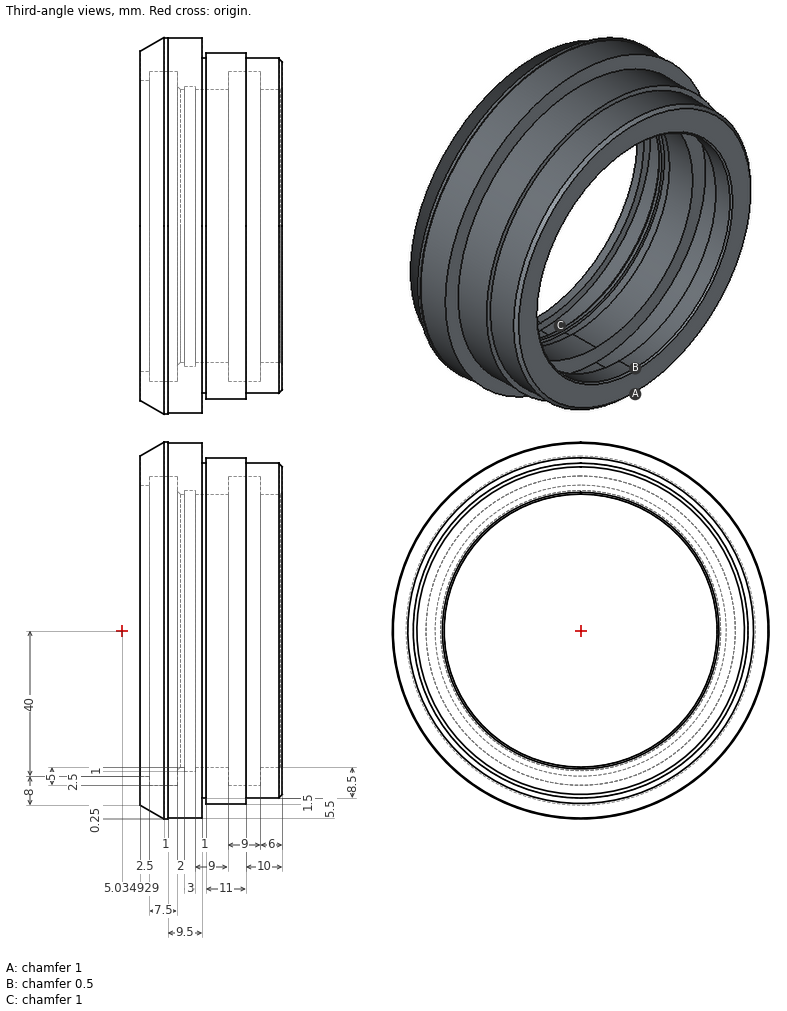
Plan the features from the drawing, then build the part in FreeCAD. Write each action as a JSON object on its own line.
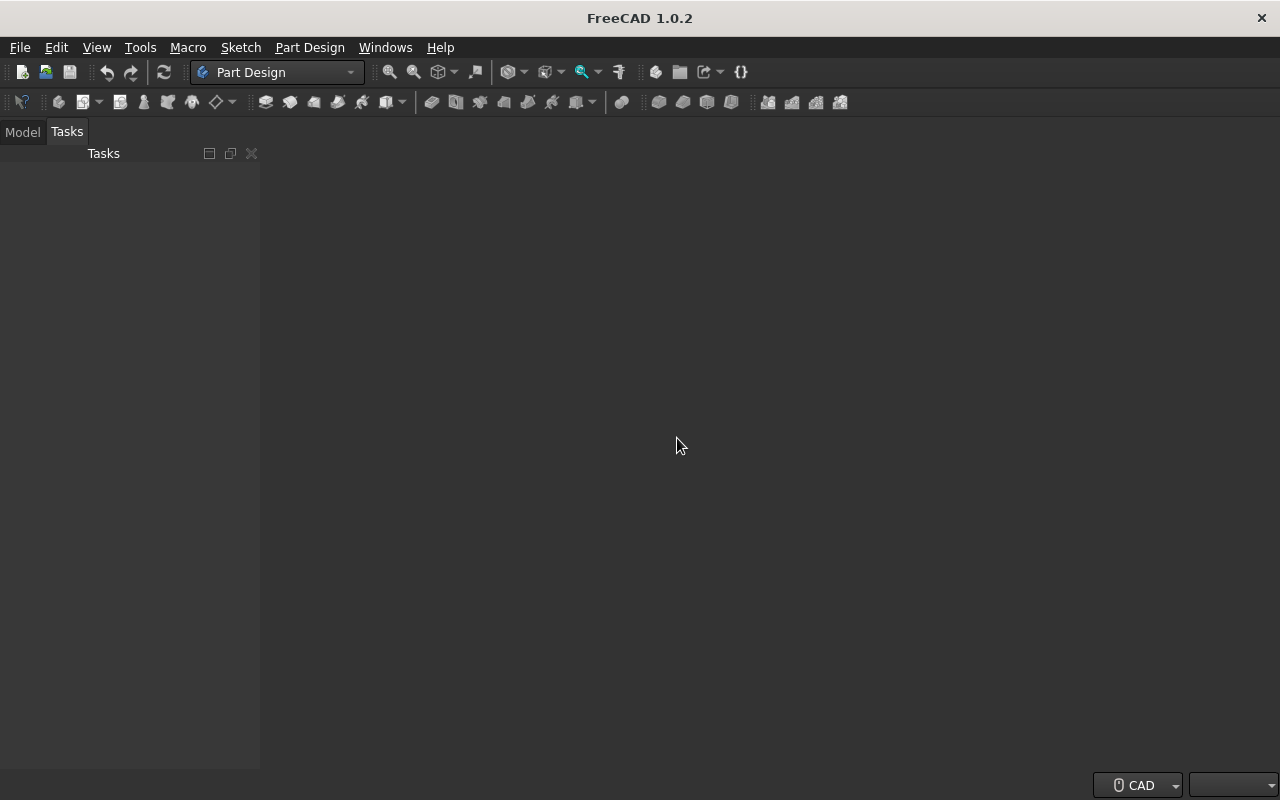
{"action": "key", "text": "ctrl+n"}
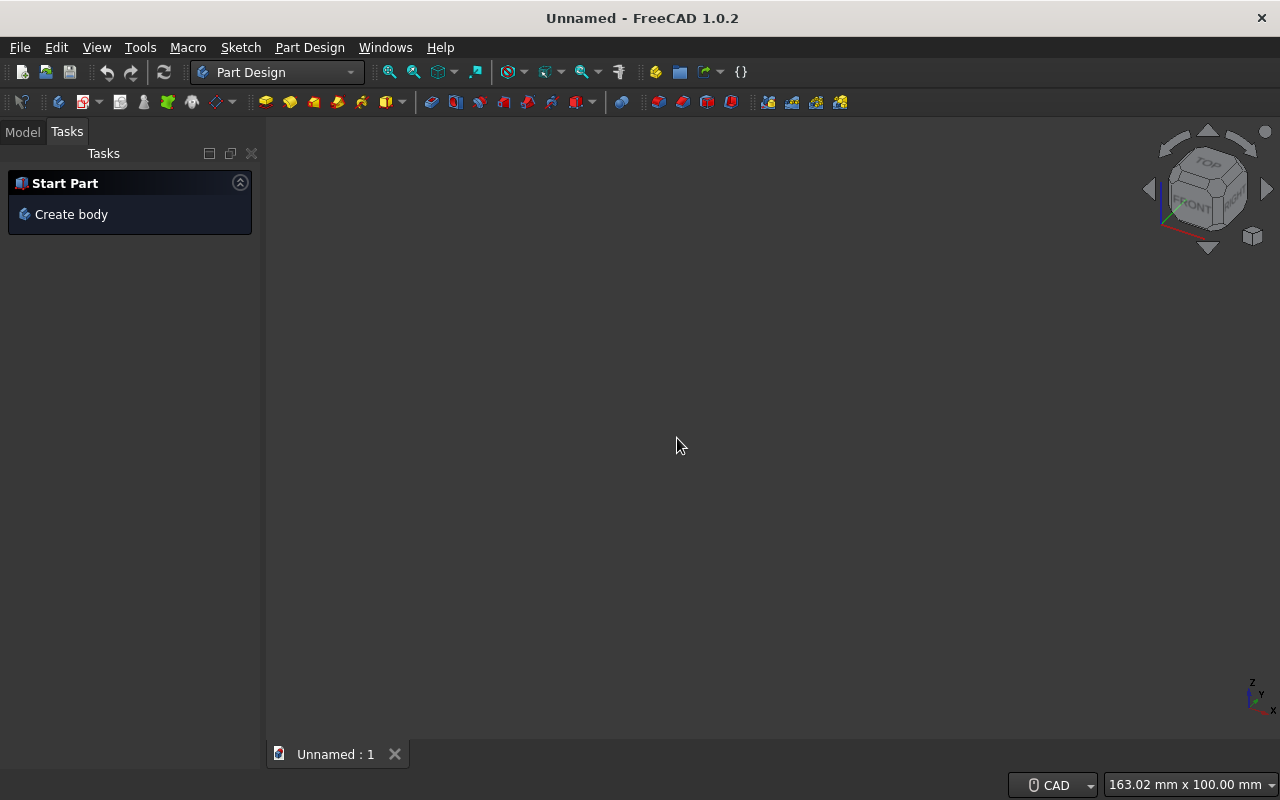
{"action": "left_click", "coordinate": [84, 102]}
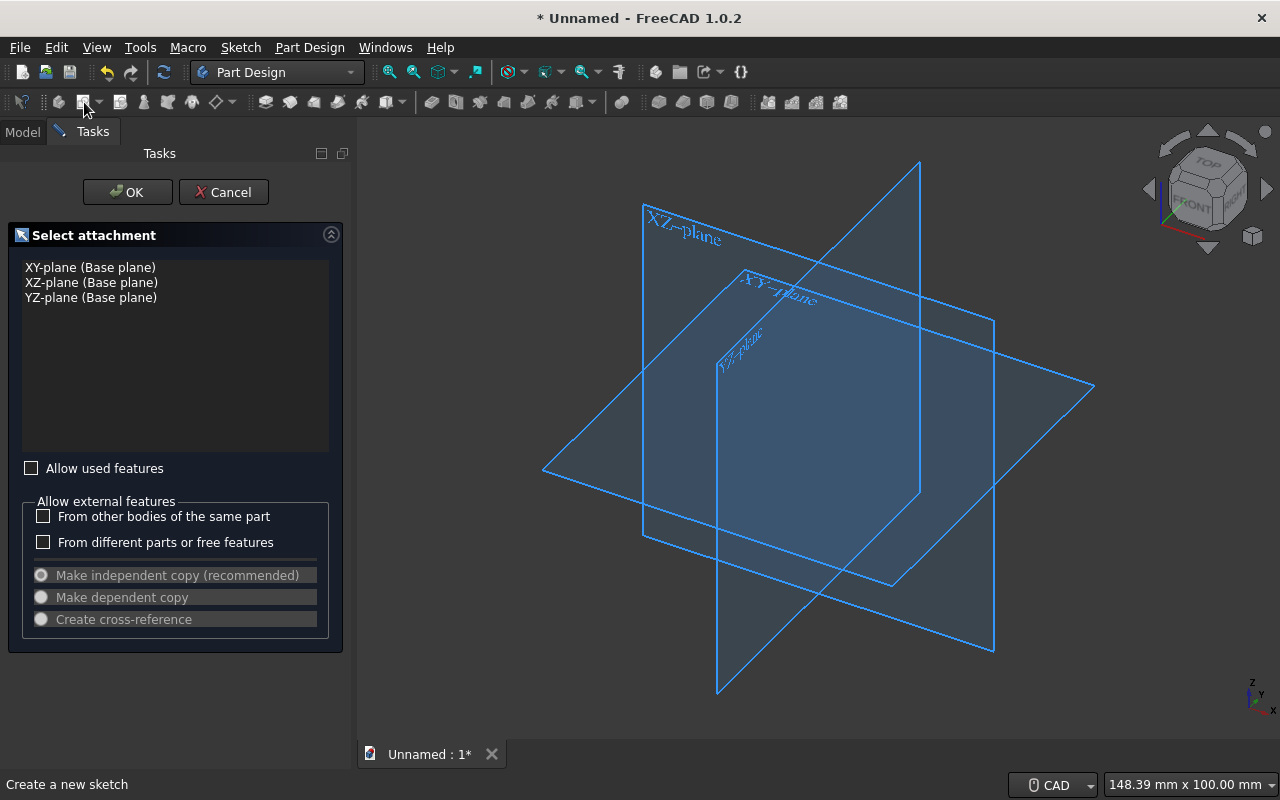
{"action": "left_click", "coordinate": [82, 282]}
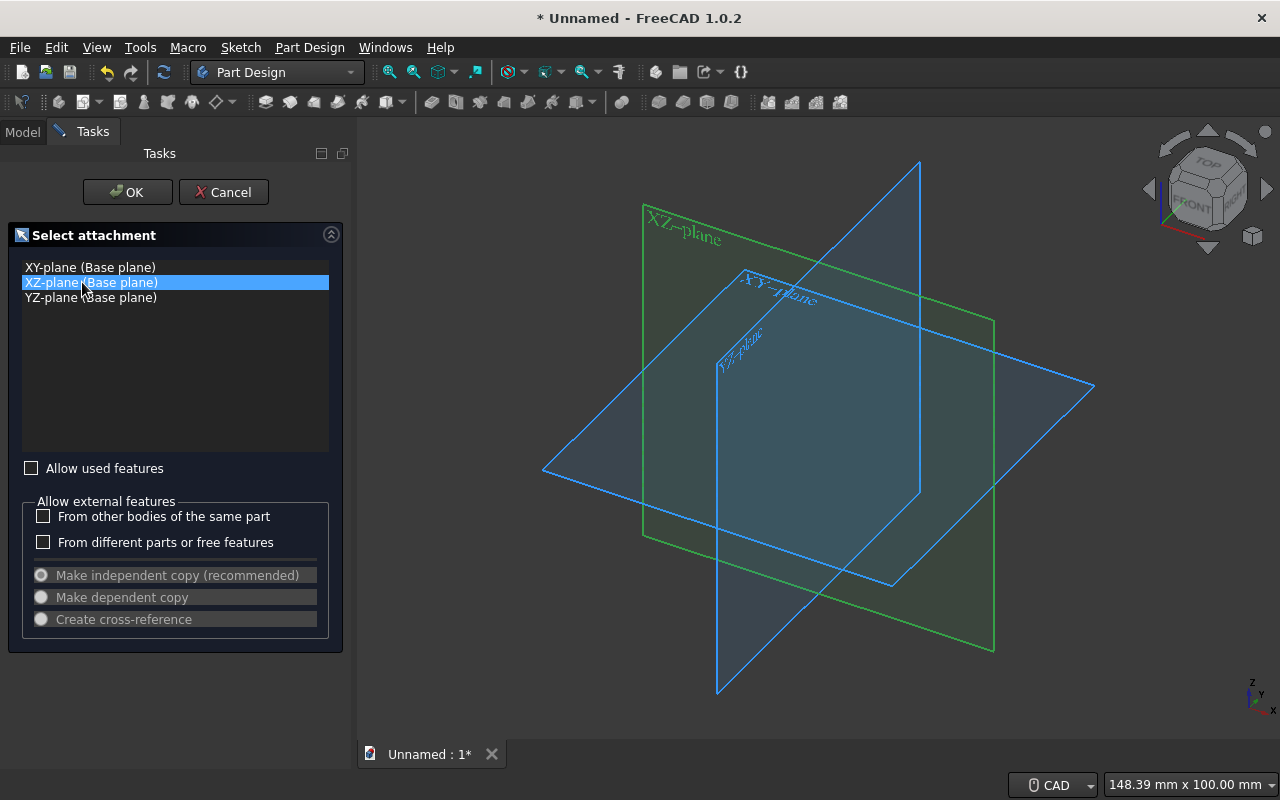
{"action": "left_click", "coordinate": [128, 192]}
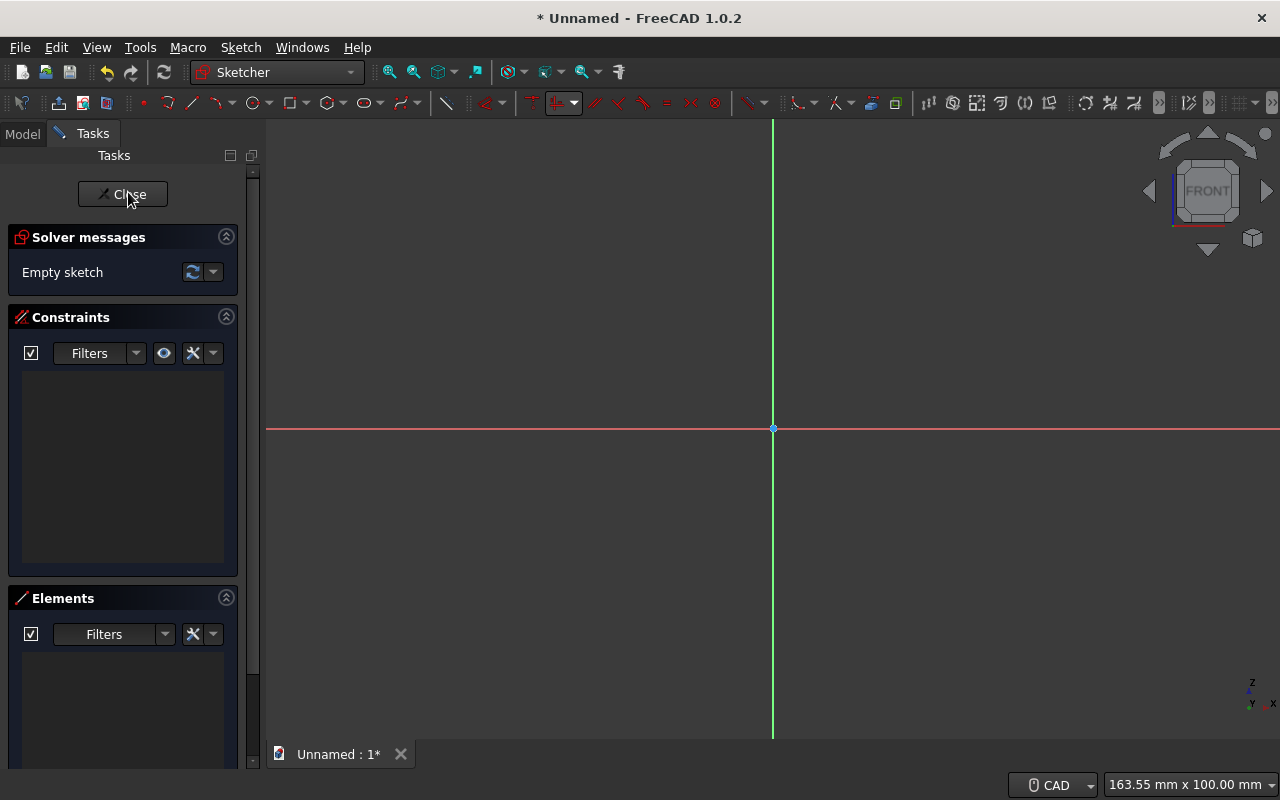
{"action": "scroll", "coordinate": [294, 147], "scroll_direction": "down", "scroll_amount": 1}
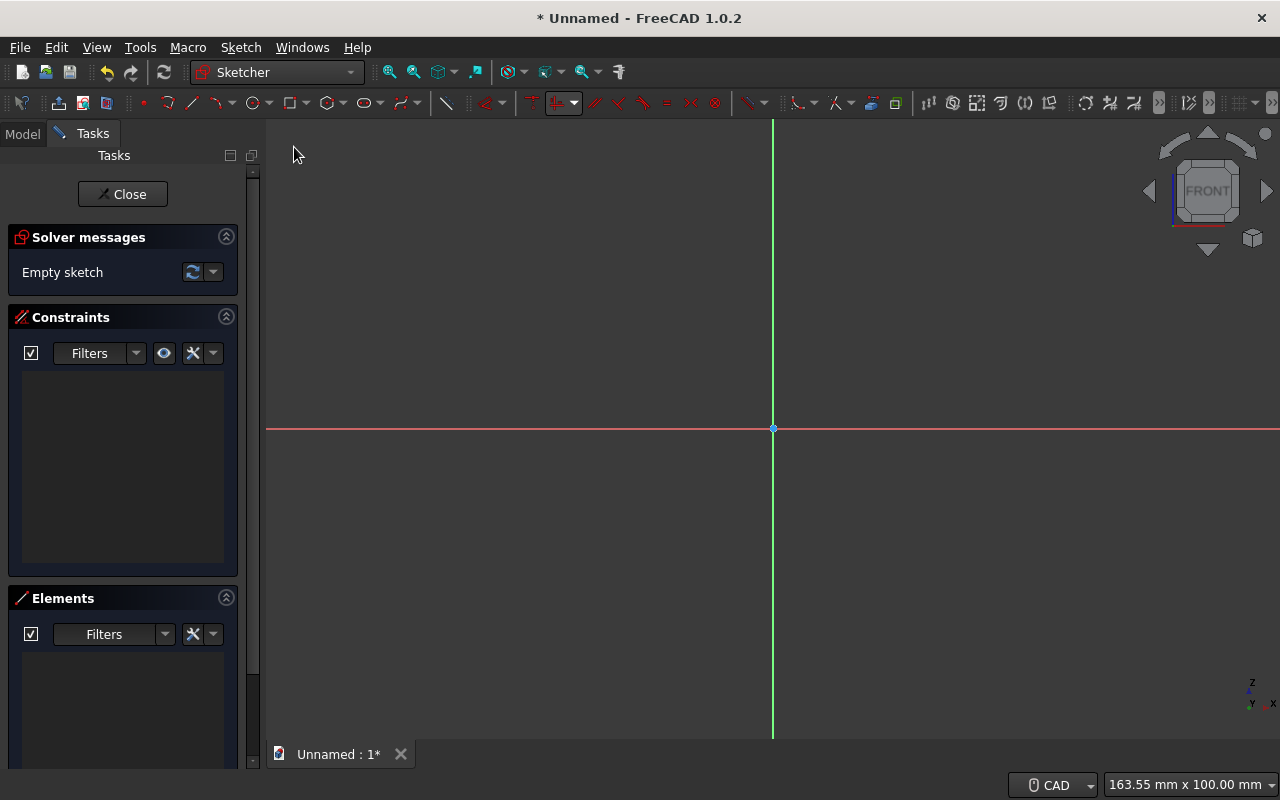
{"action": "scroll", "coordinate": [988, 672], "scroll_direction": "up", "scroll_amount": 2}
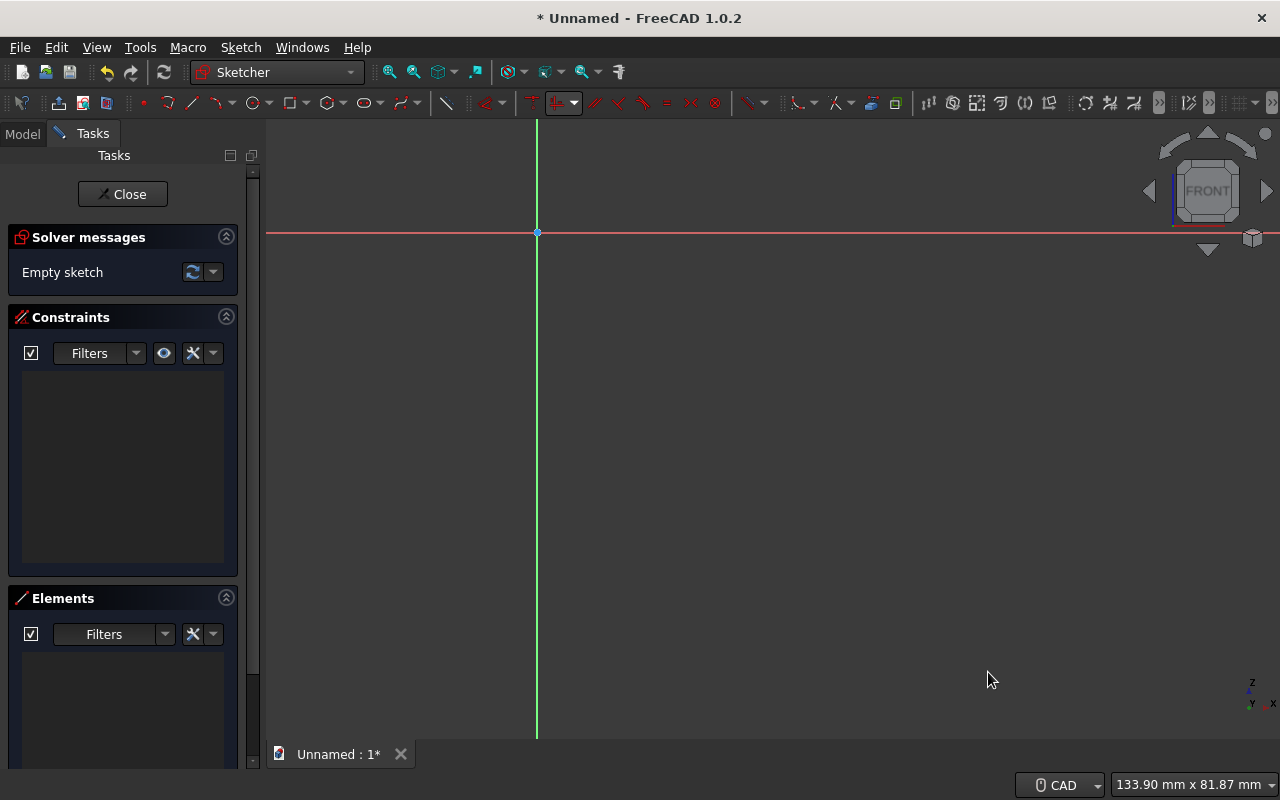
{"action": "key", "text": "g m"}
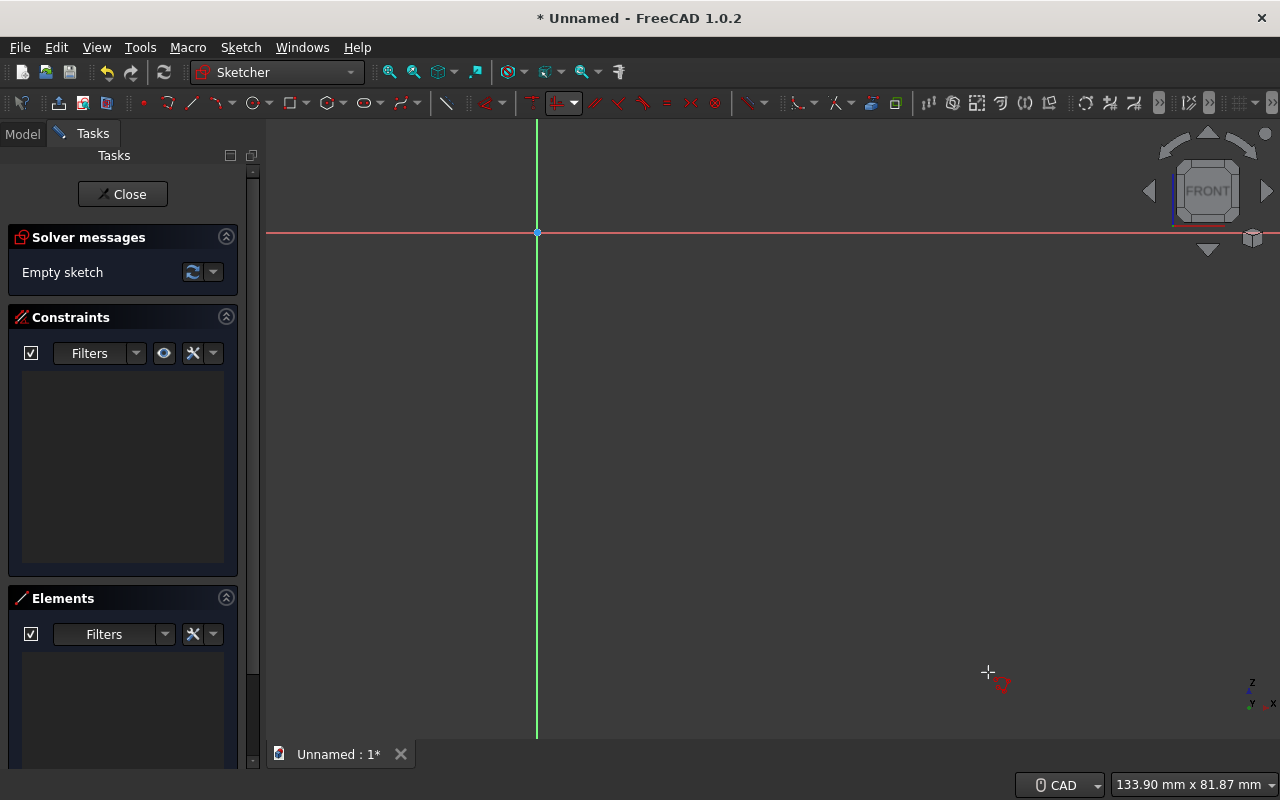
{"action": "left_click", "coordinate": [576, 536]}
{"action": "left_click", "coordinate": [594, 536]}
{"action": "left_click", "coordinate": [594, 555]}
{"action": "left_click", "coordinate": [651, 555]}
{"action": "left_click", "coordinate": [651, 517]}
{"action": "left_click", "coordinate": [666, 517]}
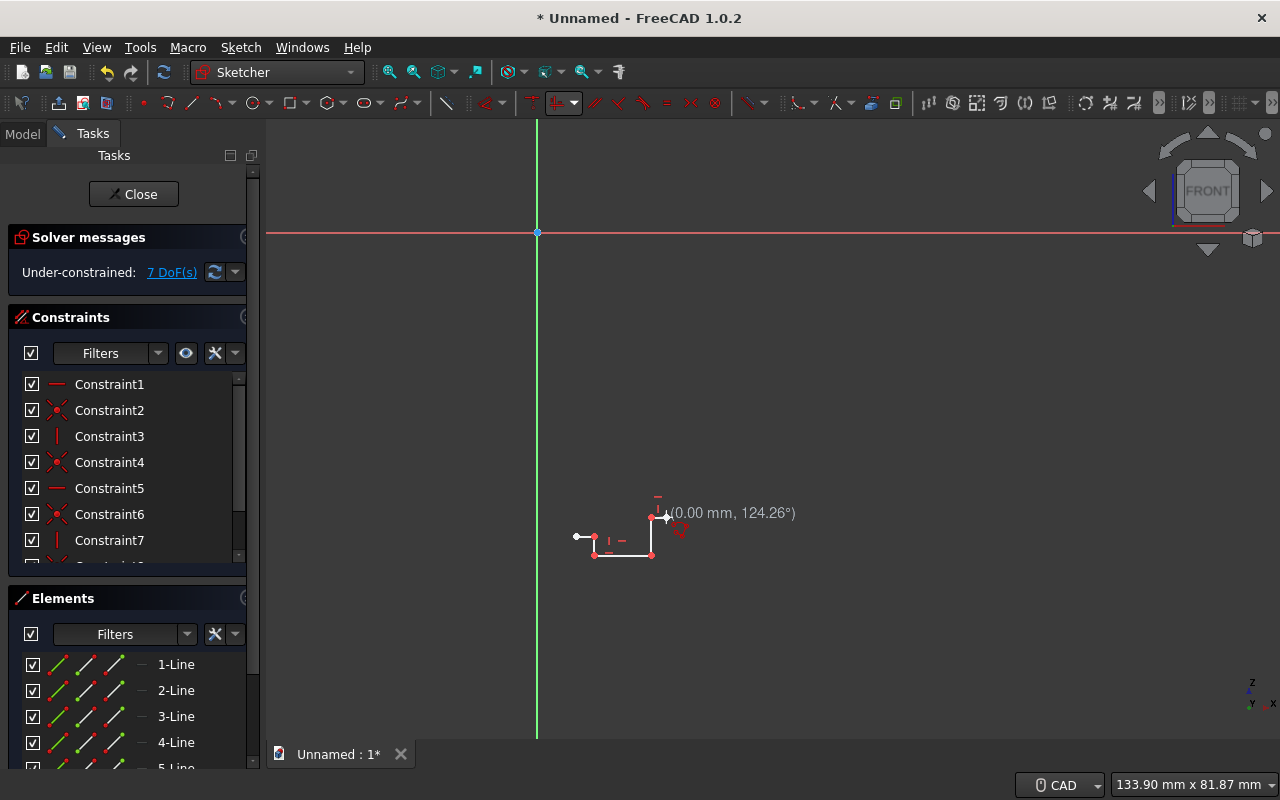
{"action": "scroll", "coordinate": [666, 524], "scroll_direction": "up", "scroll_amount": 4}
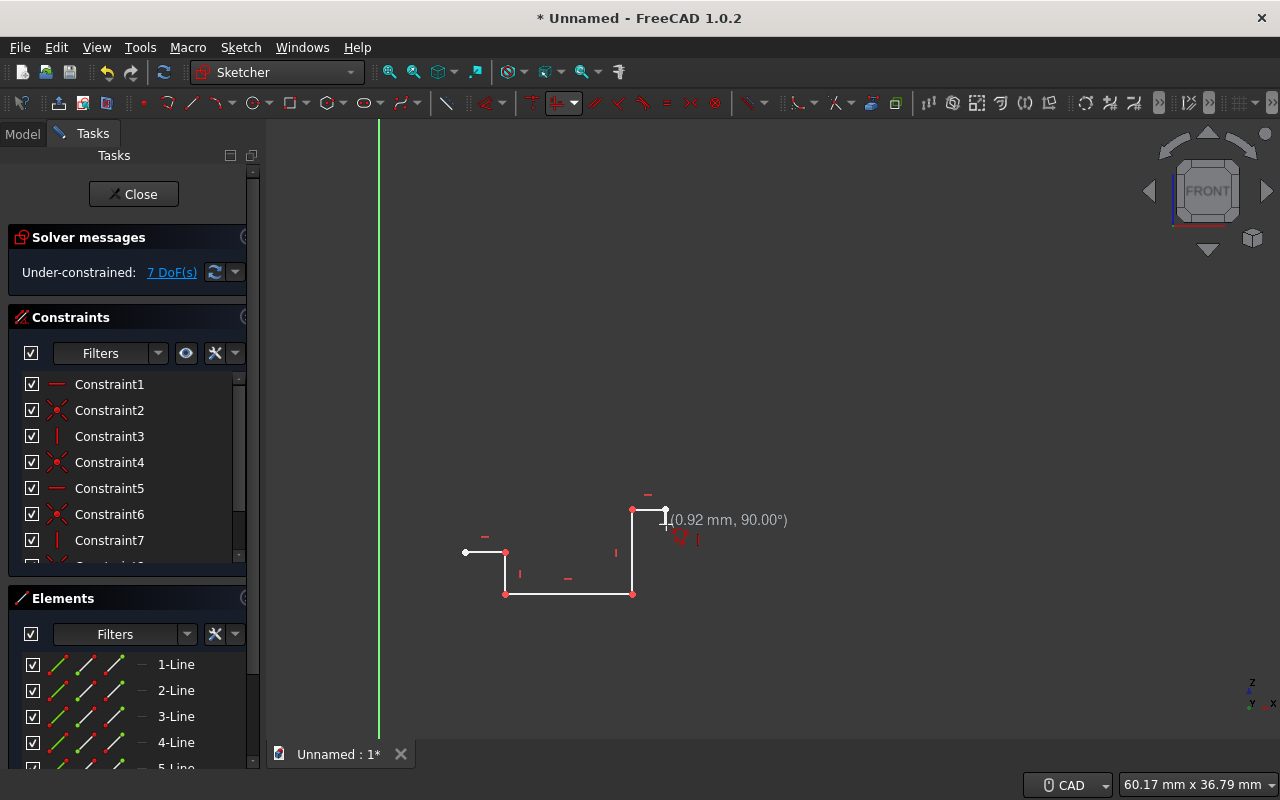
{"action": "left_click", "coordinate": [666, 524]}
{"action": "left_click", "coordinate": [717, 524]}
{"action": "left_click", "coordinate": [717, 507]}
{"action": "left_click", "coordinate": [869, 507]}
{"action": "left_click", "coordinate": [869, 591]}
{"action": "left_click", "coordinate": [1020, 591]}
{"action": "left_click", "coordinate": [1020, 507]}